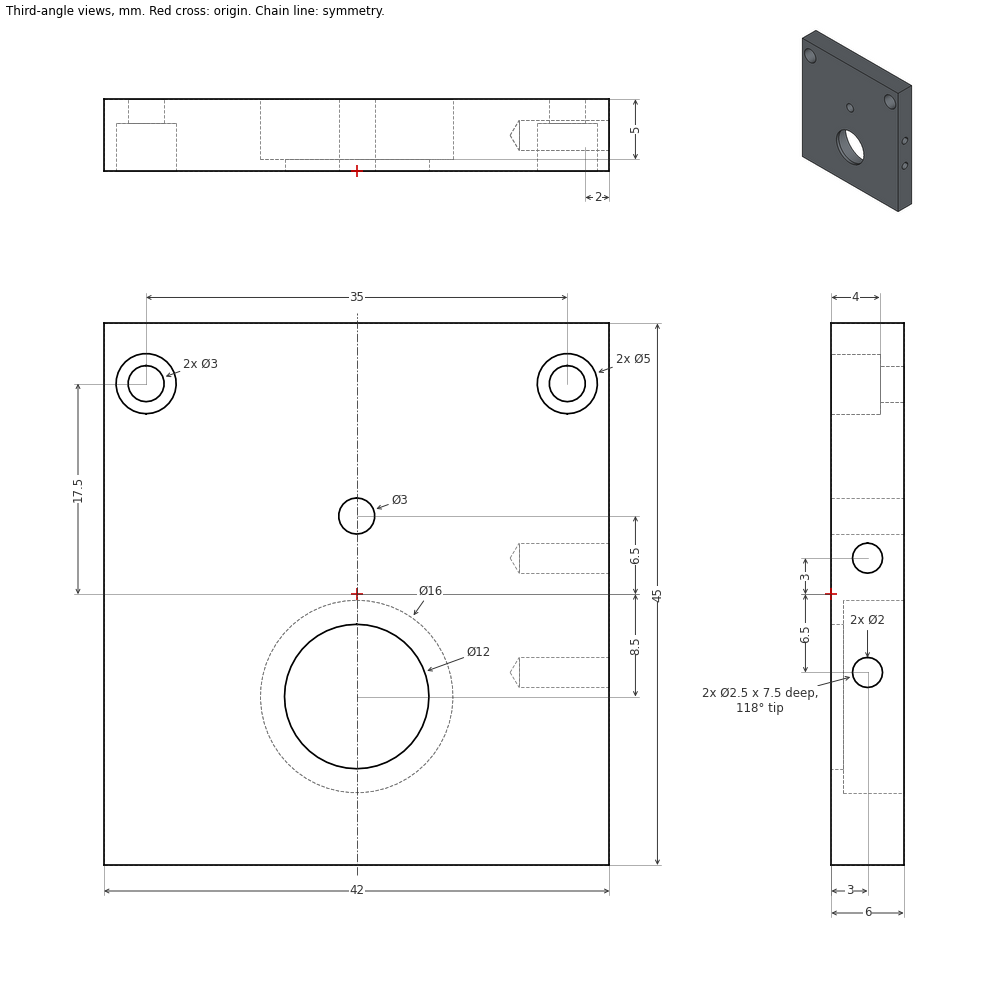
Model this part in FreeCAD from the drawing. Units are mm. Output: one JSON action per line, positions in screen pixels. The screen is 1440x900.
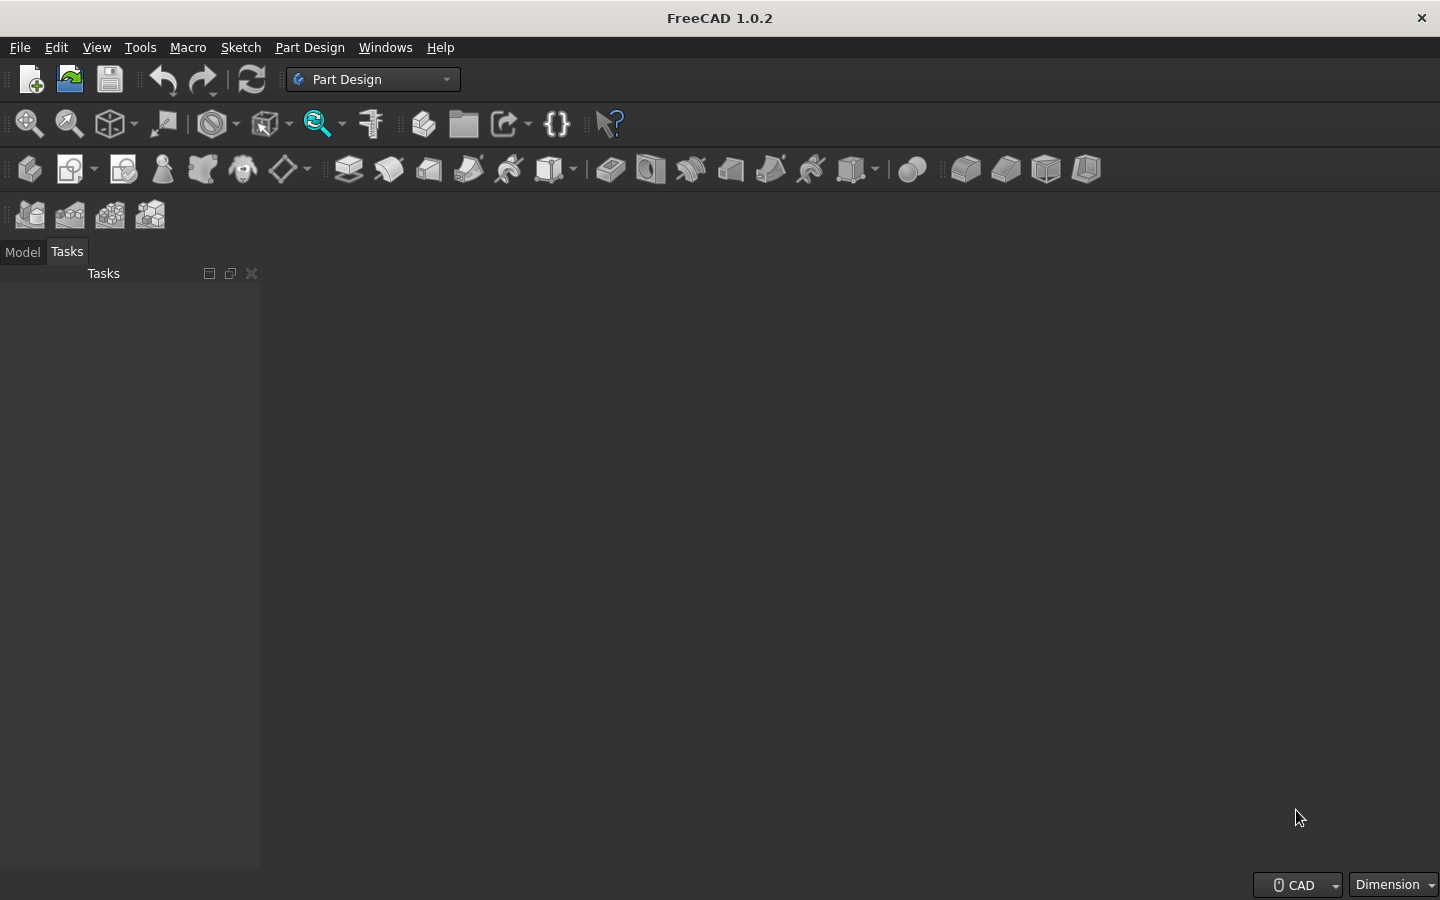
{"action": "key", "text": "ctrl+n"}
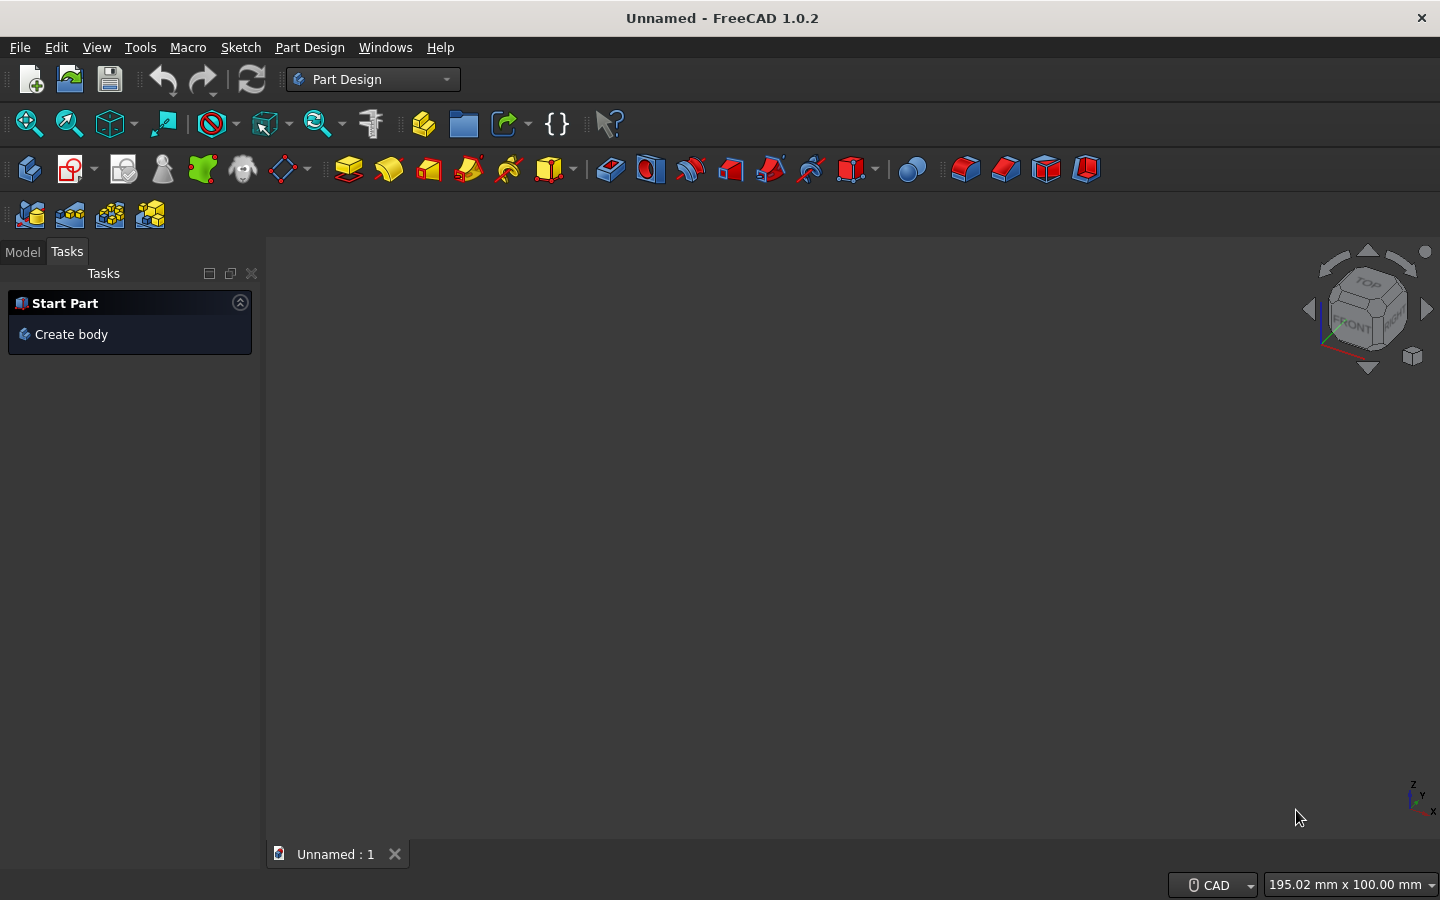
{"action": "left_click", "coordinate": [70, 170]}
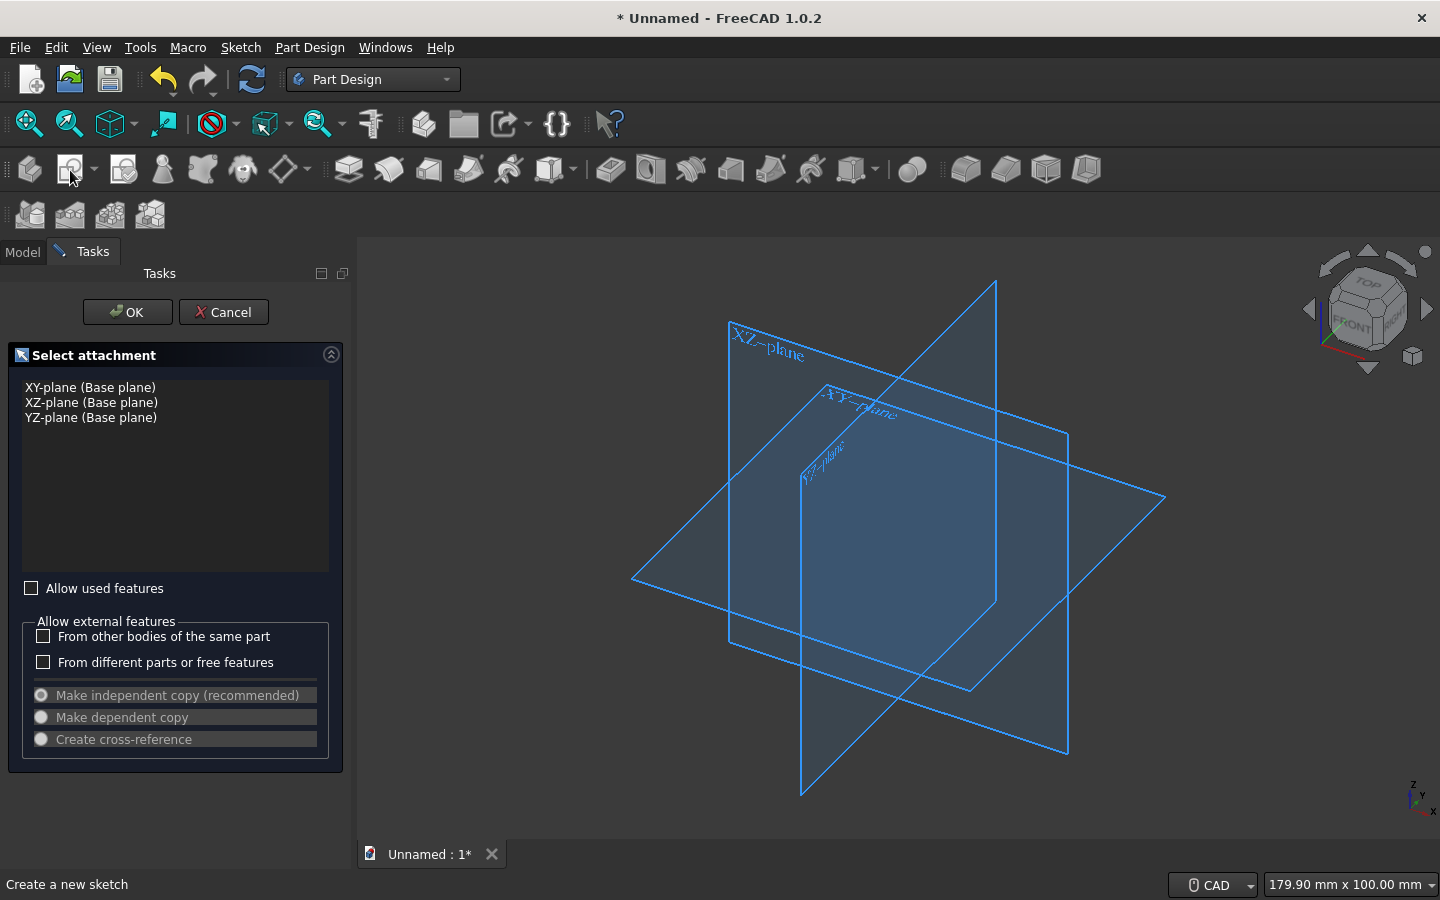
{"action": "left_click", "coordinate": [82, 402]}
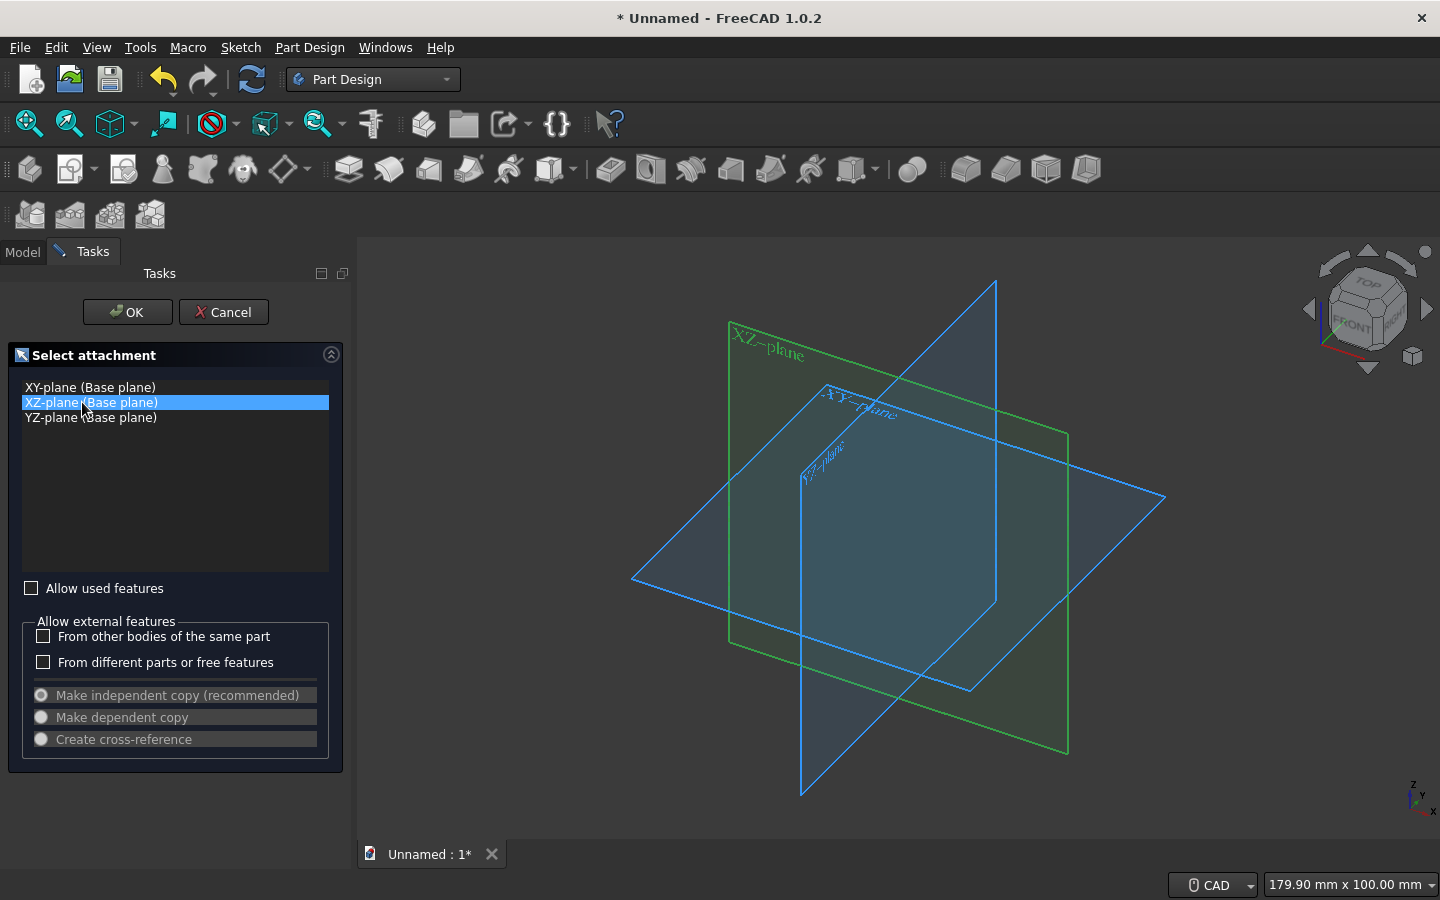
{"action": "left_click", "coordinate": [128, 312]}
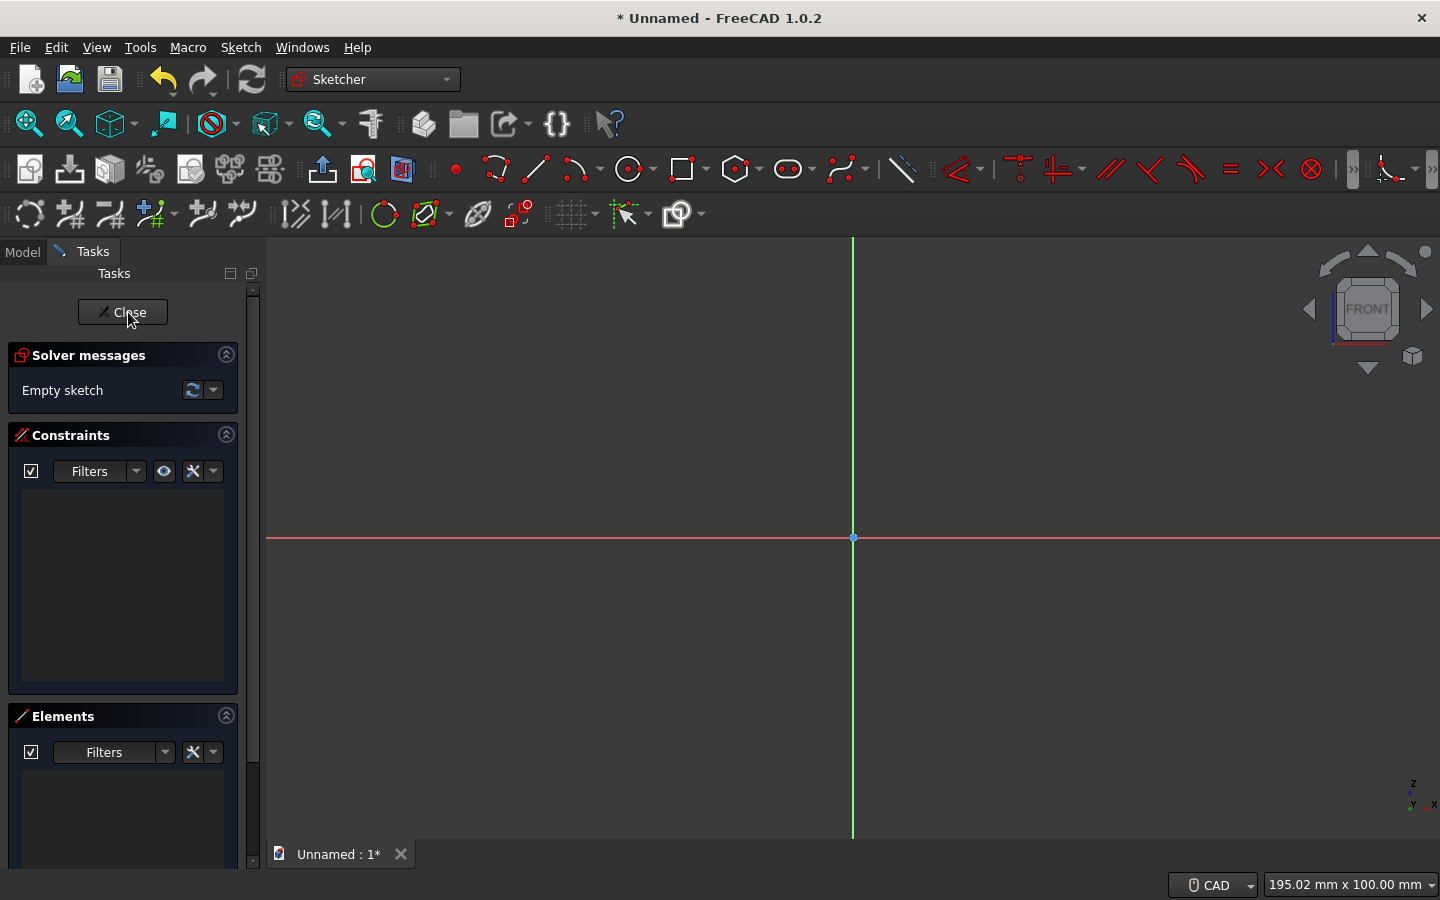
{"action": "scroll", "coordinate": [992, 538], "scroll_direction": "up", "scroll_amount": 2}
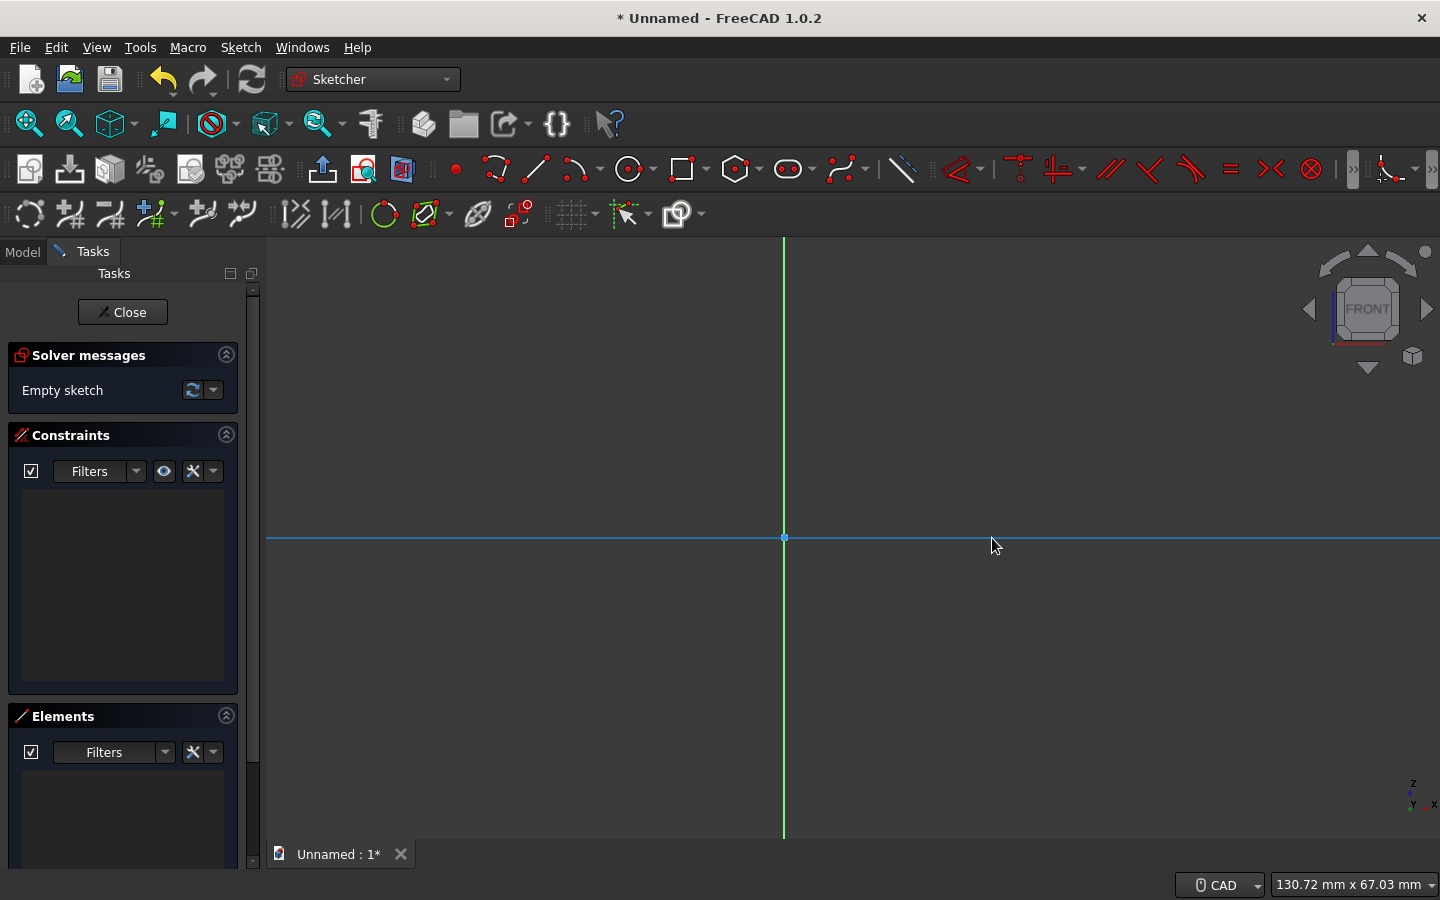
{"action": "key", "text": "g v"}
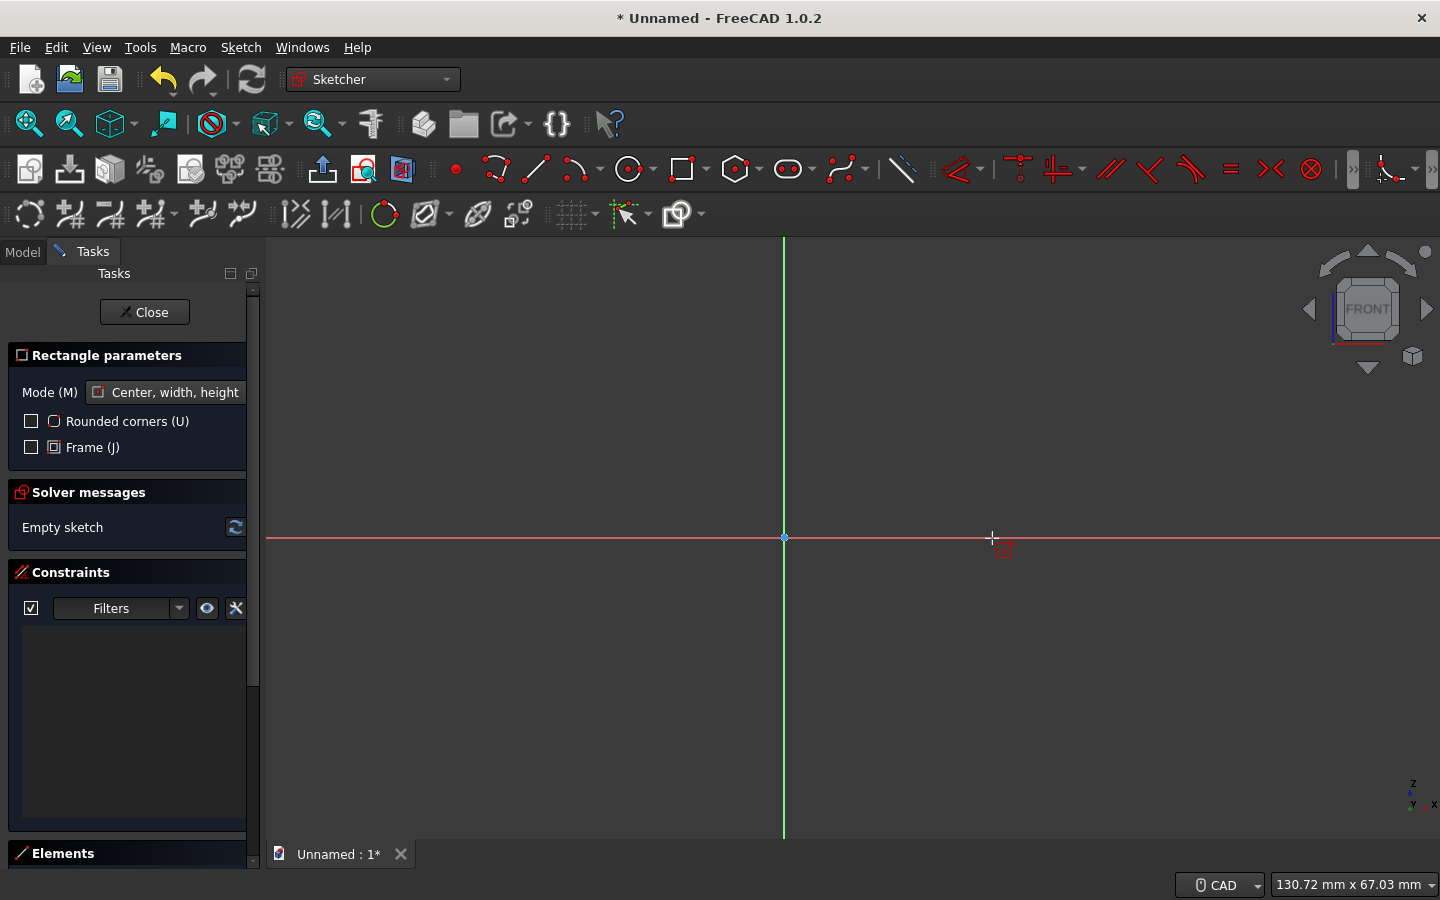
{"action": "left_click", "coordinate": [784, 538]}
{"action": "mouse_move", "coordinate": [973, 336]}